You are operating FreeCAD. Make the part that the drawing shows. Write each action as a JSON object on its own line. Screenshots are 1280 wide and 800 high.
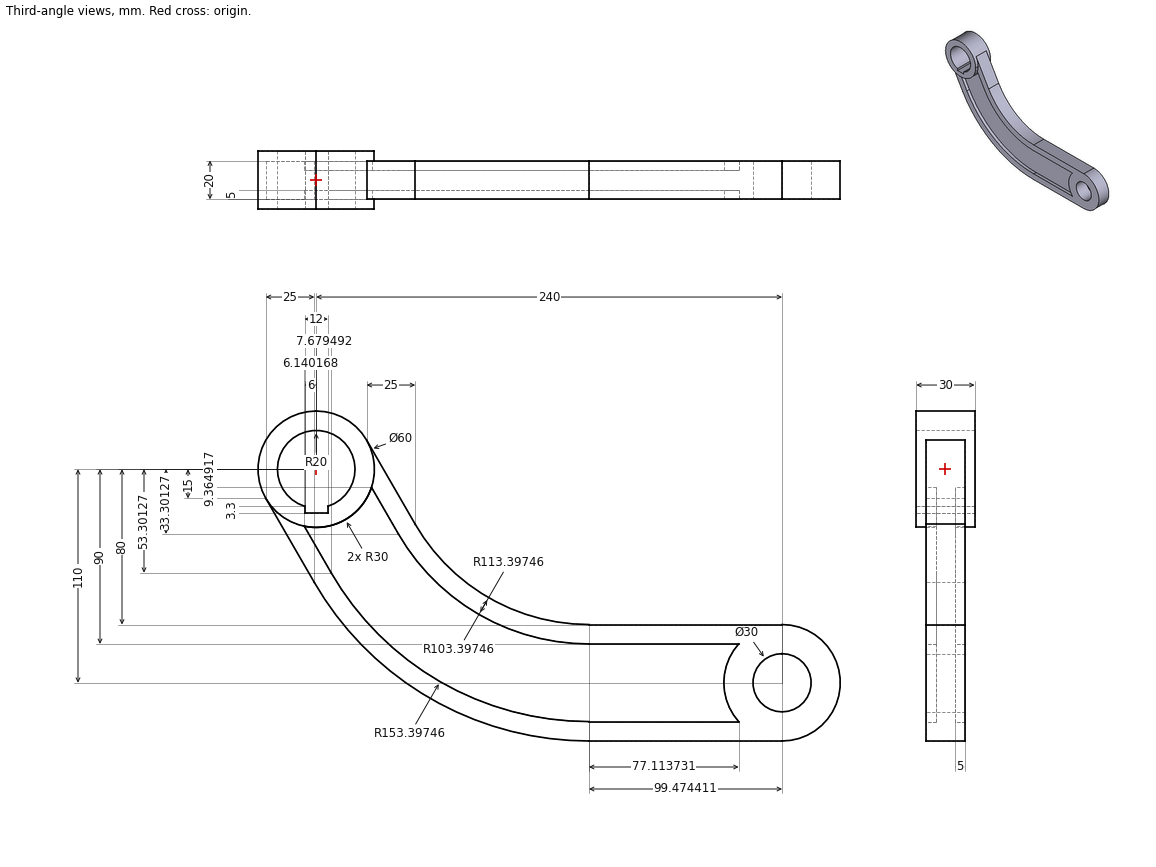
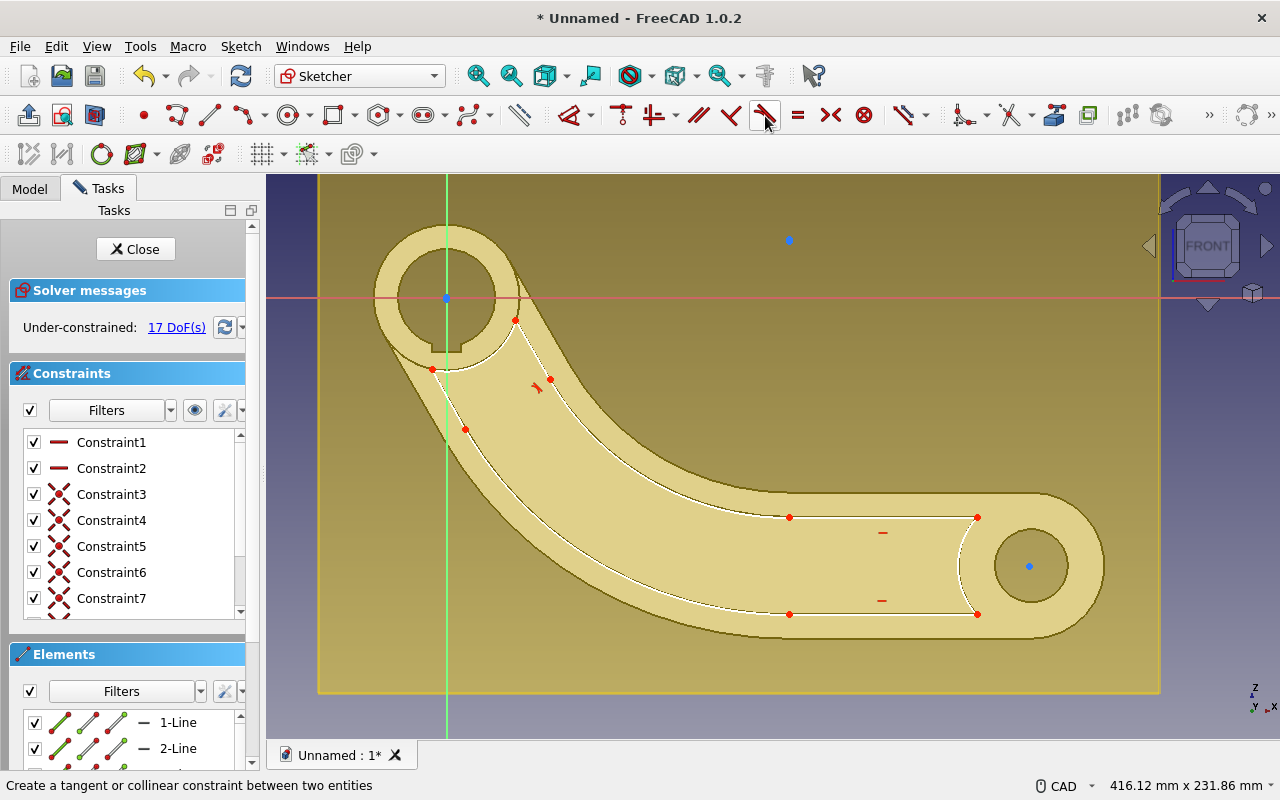
{"action": "left_click", "coordinate": [445, 394]}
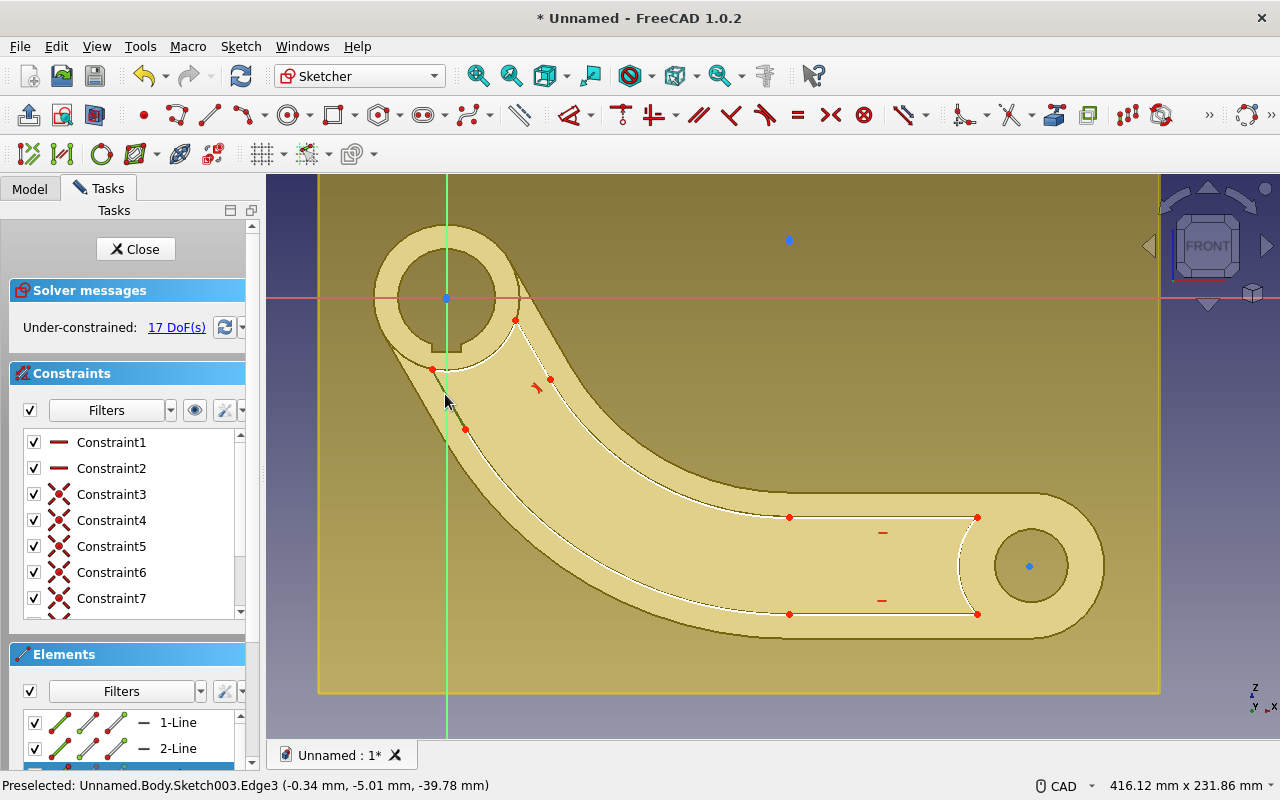
{"action": "left_click", "coordinate": [539, 519]}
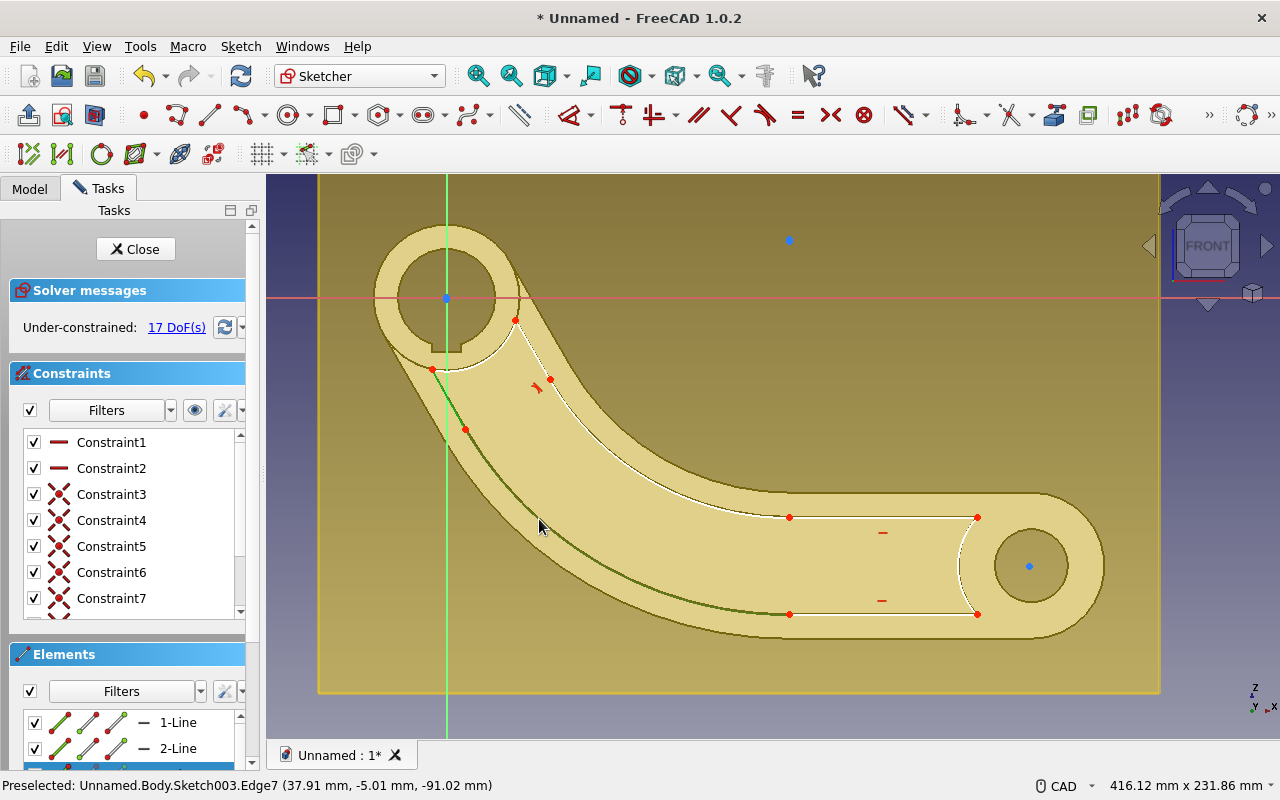
{"action": "left_click", "coordinate": [765, 116]}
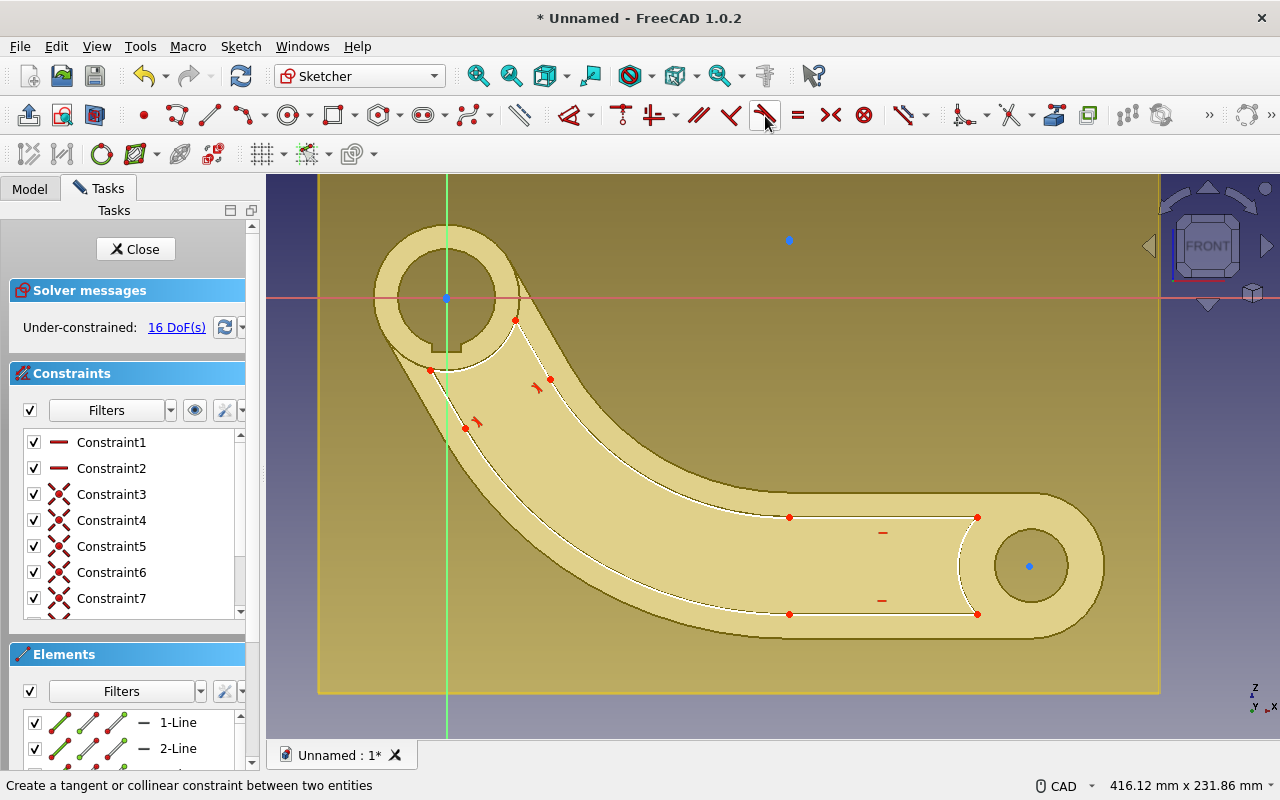
{"action": "left_click", "coordinate": [604, 447]}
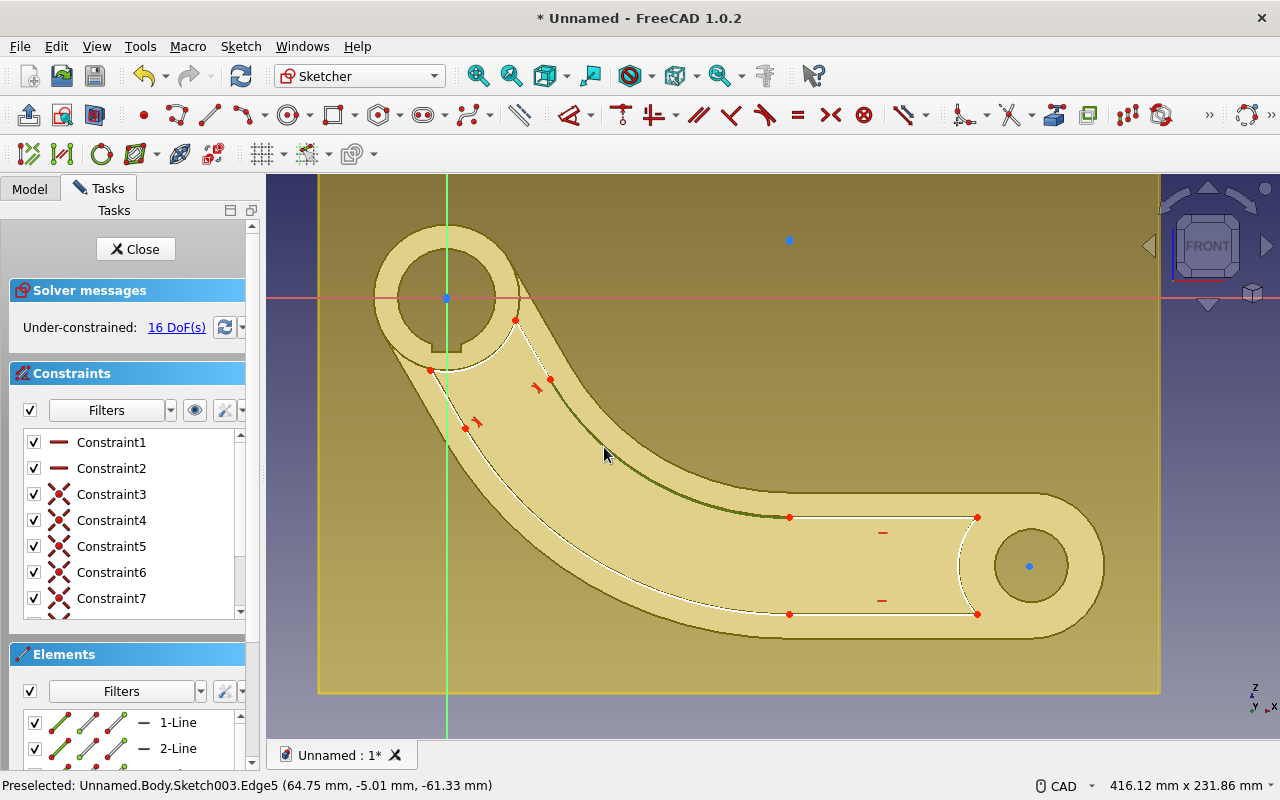
{"action": "left_click", "coordinate": [539, 519]}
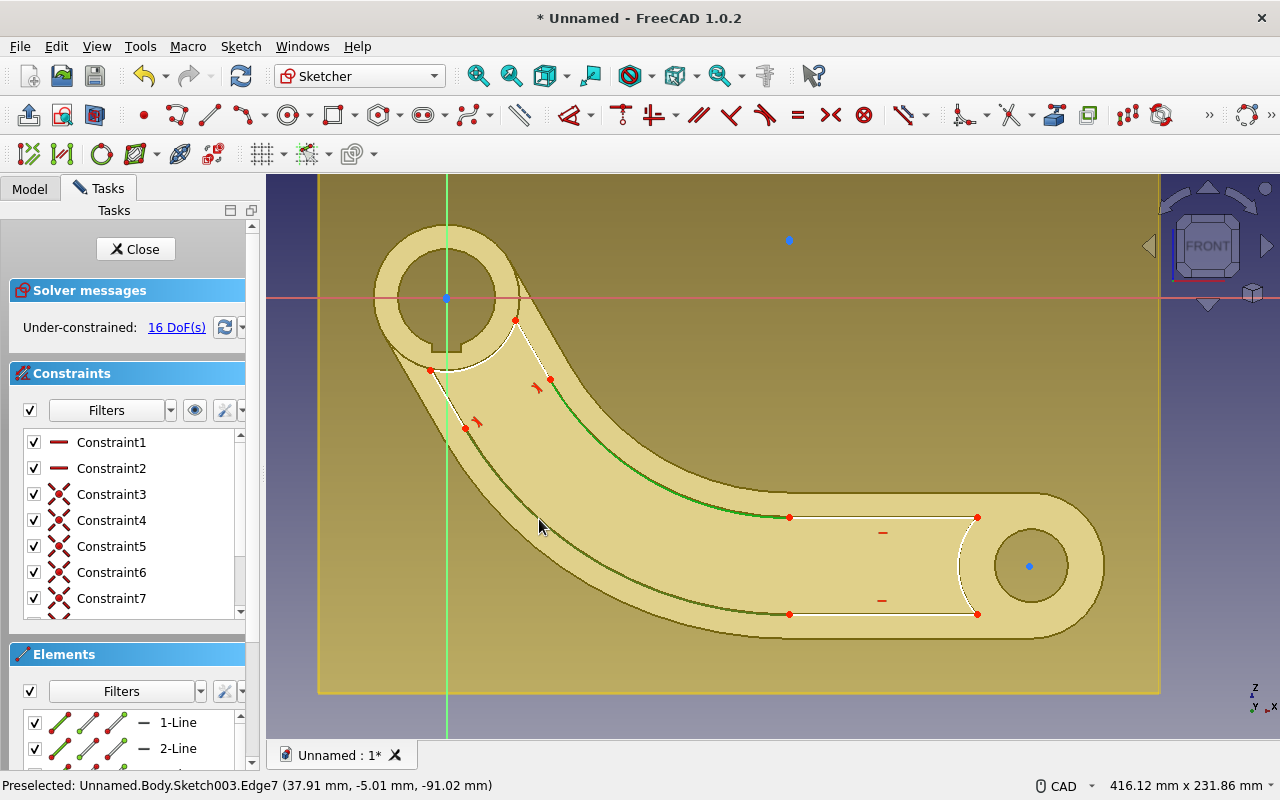
{"action": "left_click", "coordinate": [621, 116]}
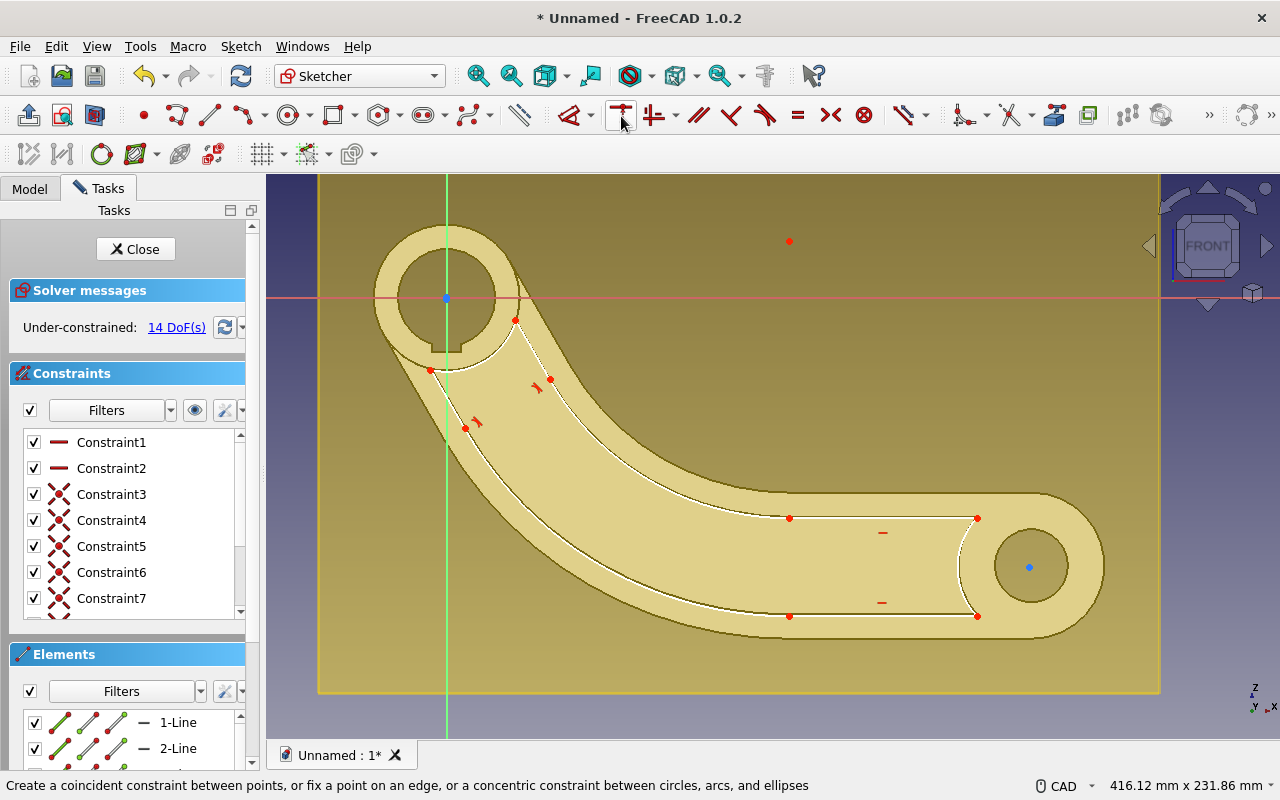
{"action": "left_click_drag", "start_coordinate": [437, 288], "coordinate": [457, 309]}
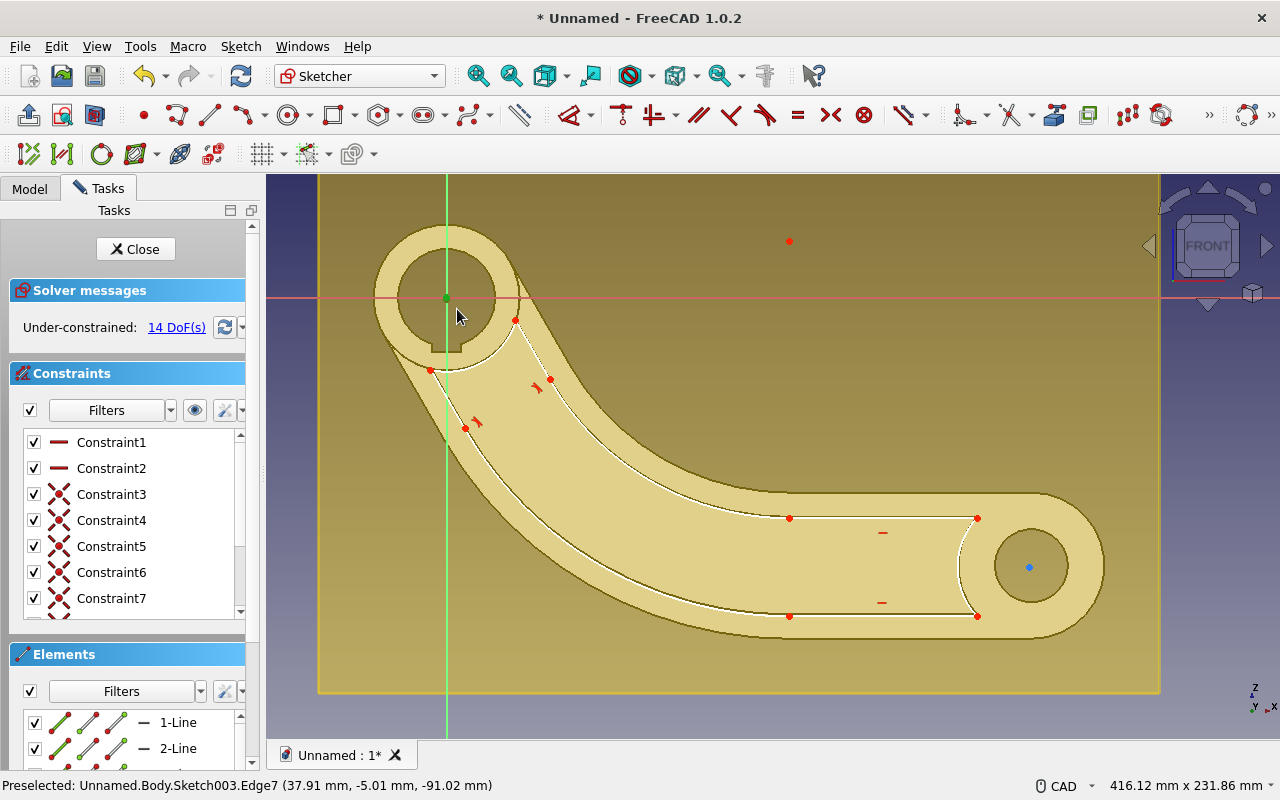
{"action": "key", "text": "c"}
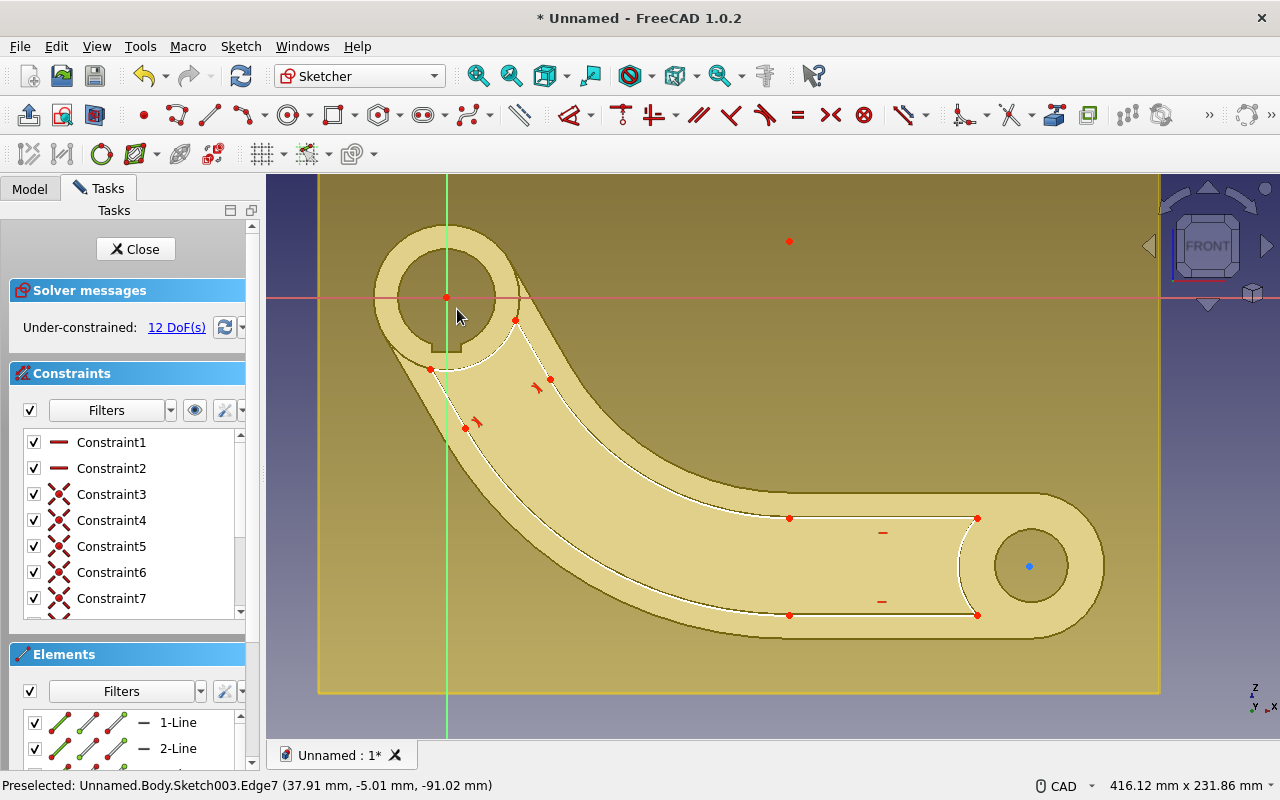
{"action": "left_click", "coordinate": [463, 369]}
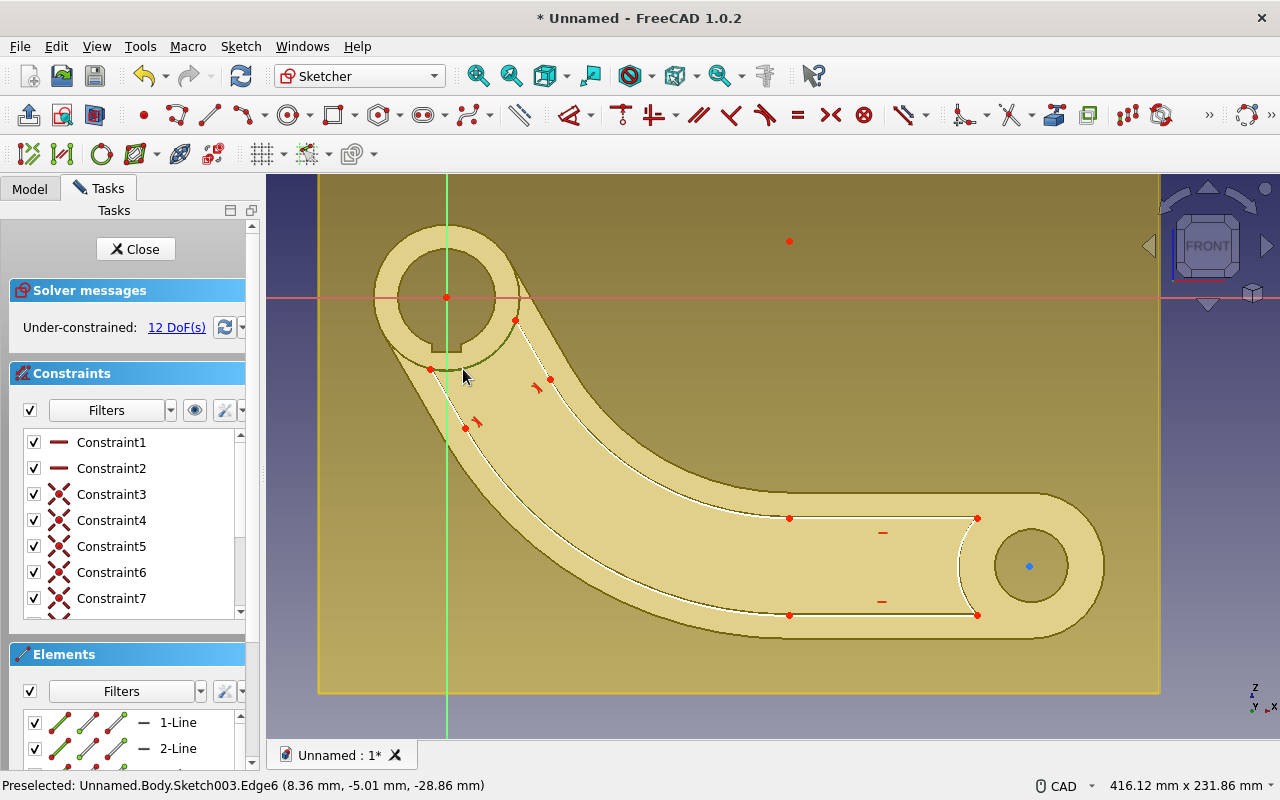
{"action": "left_click", "coordinate": [961, 546]}